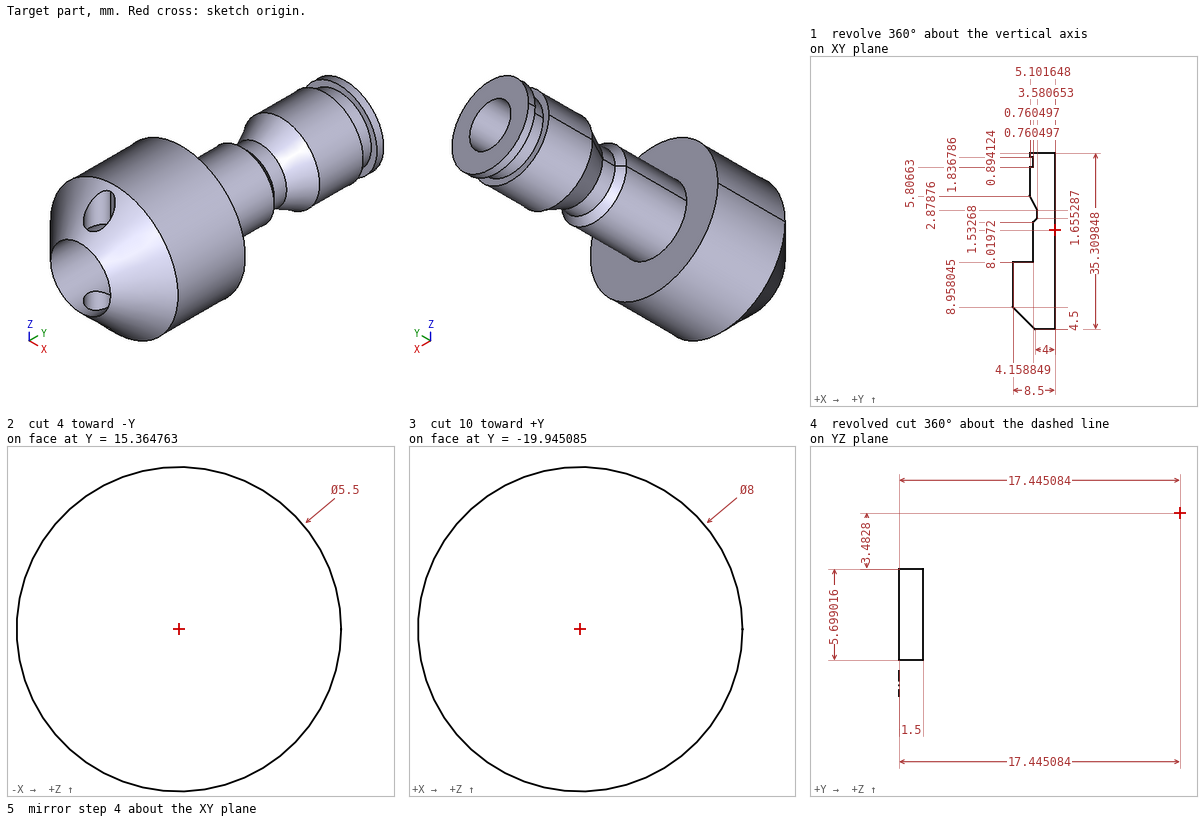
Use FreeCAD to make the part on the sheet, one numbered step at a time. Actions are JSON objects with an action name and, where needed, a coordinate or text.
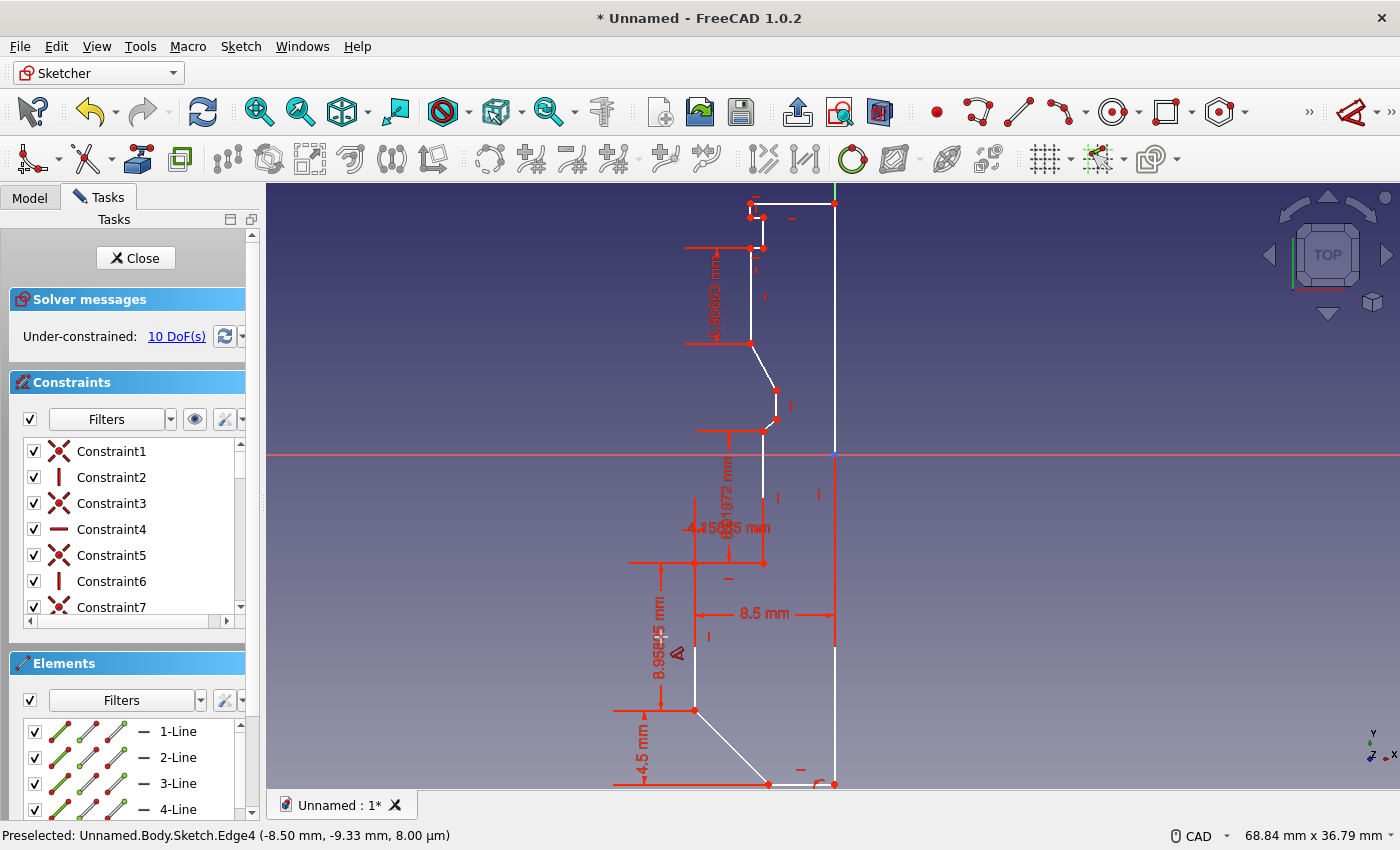
{"action": "scroll", "coordinate": [764, 472], "scroll_direction": "down", "scroll_amount": 2}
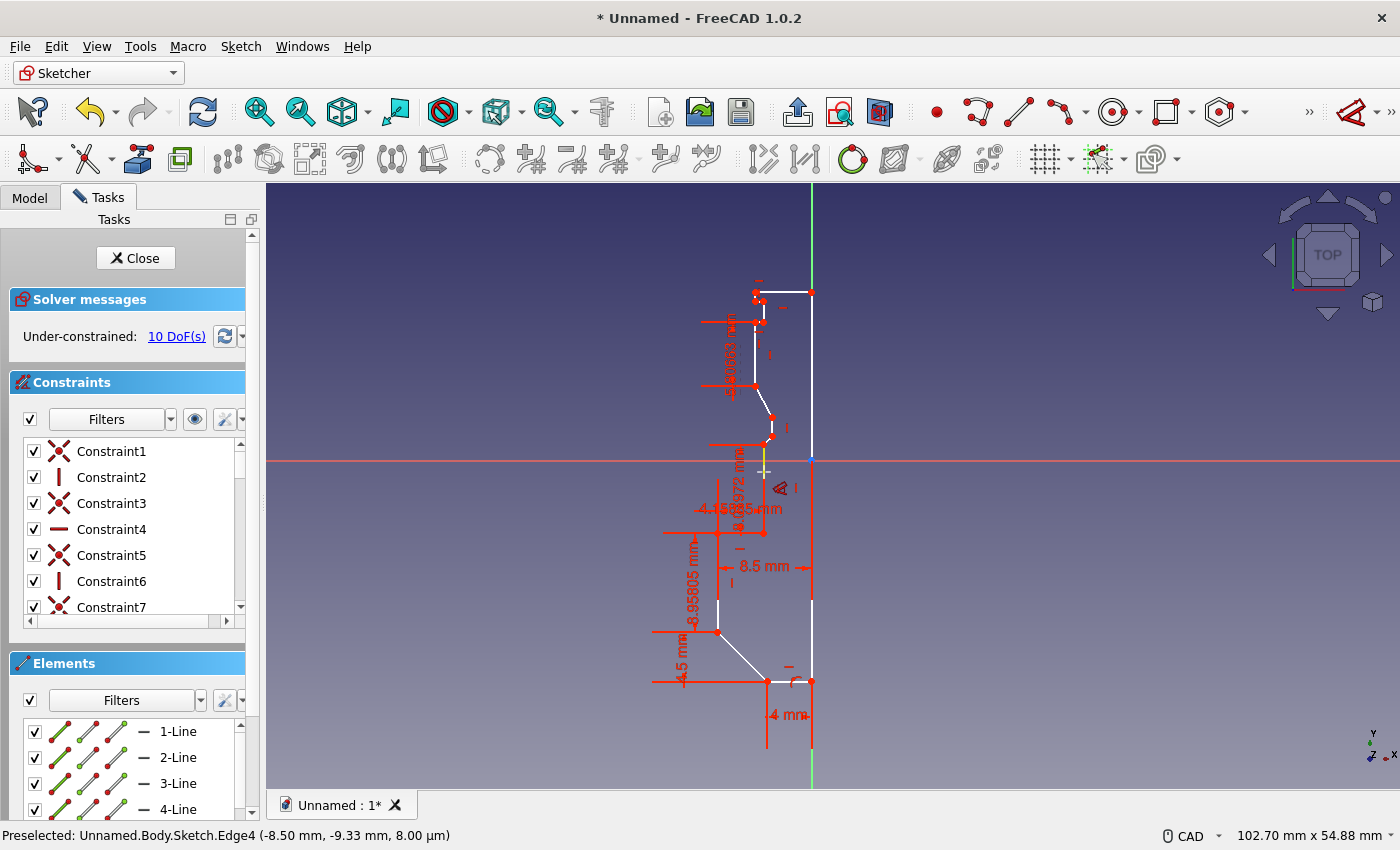
{"action": "left_click", "coordinate": [795, 292]}
{"action": "left_click", "coordinate": [783, 258]}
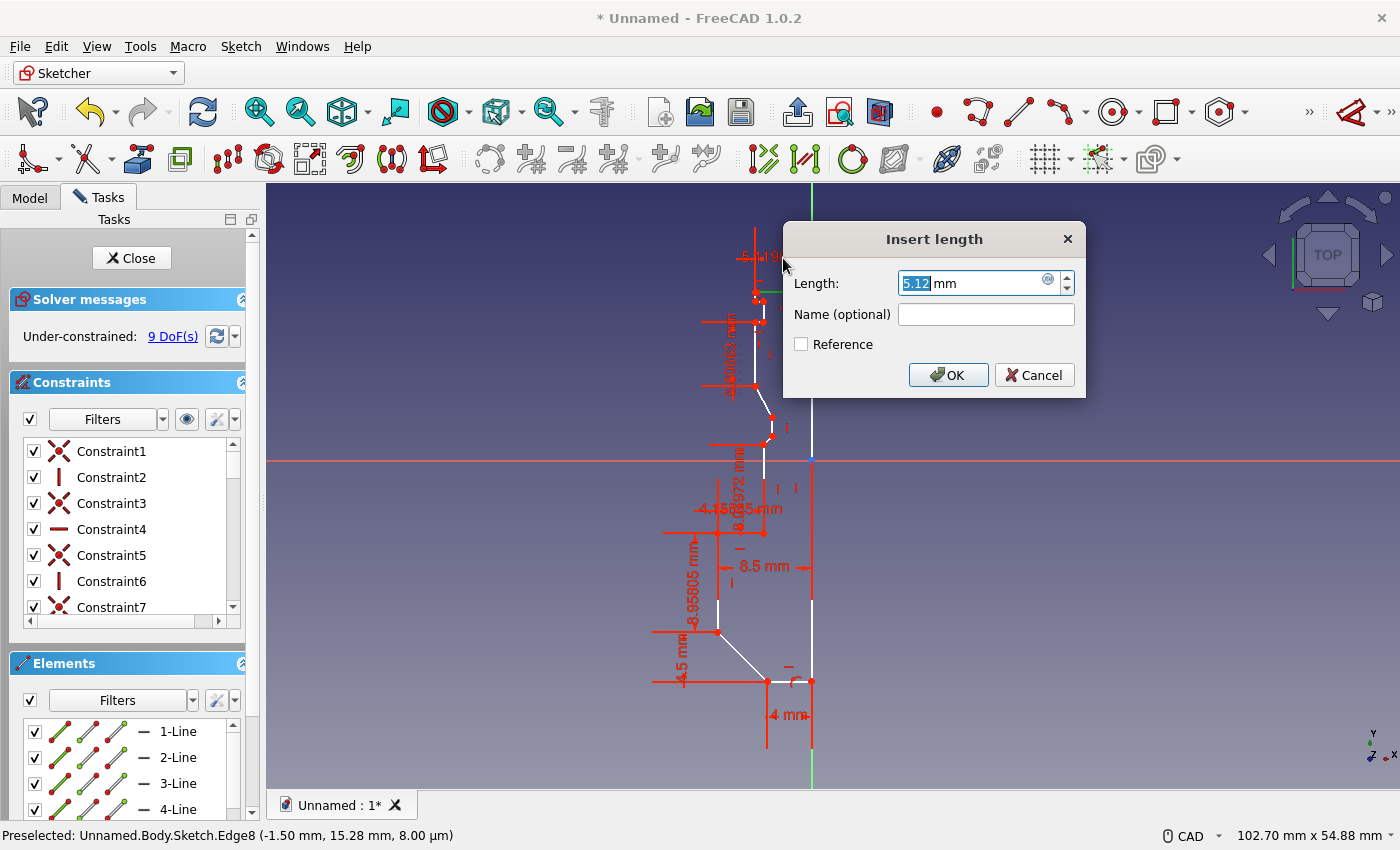
{"action": "type", "text": "5.101648"}
{"action": "key", "text": "Return"}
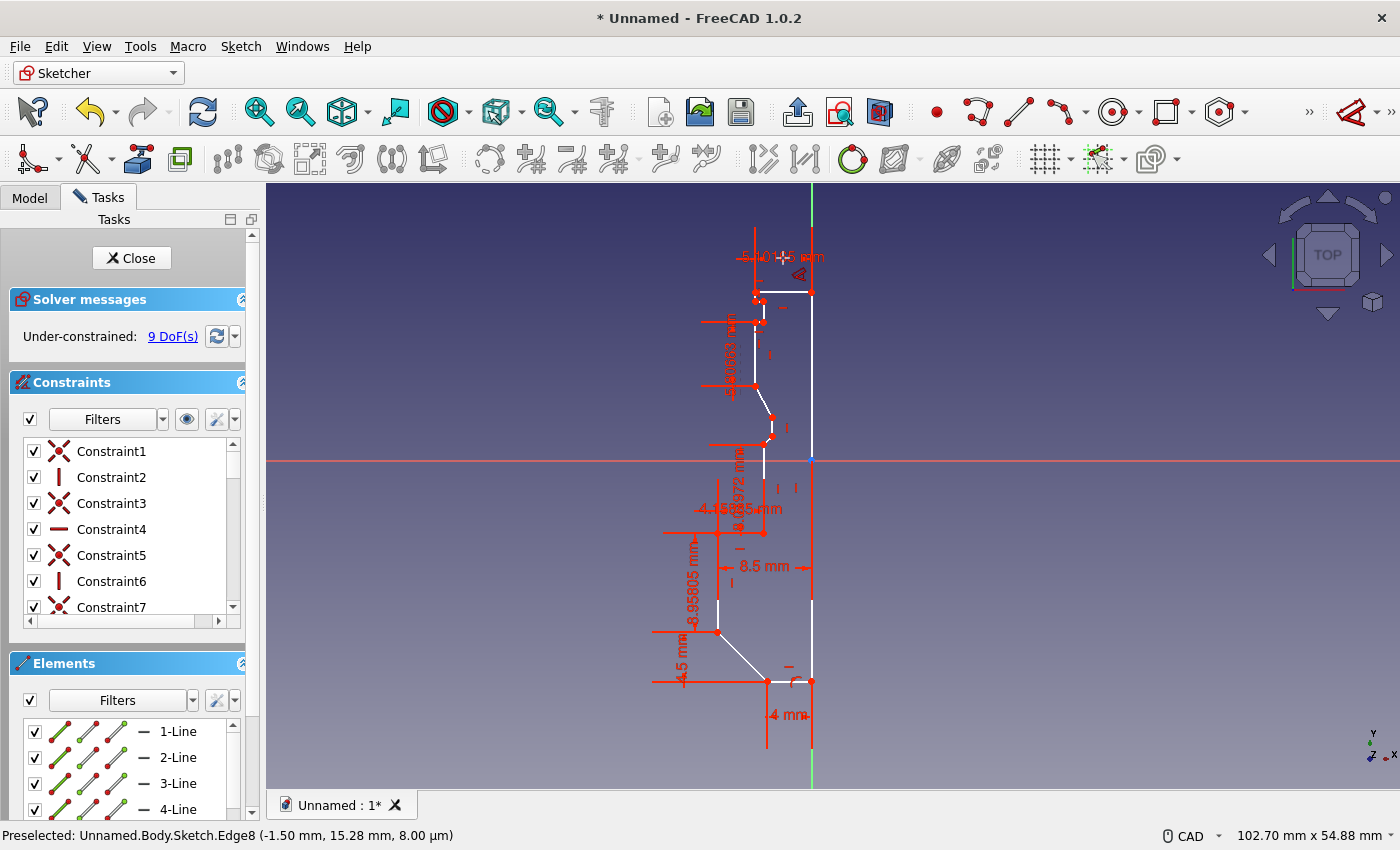
{"action": "scroll", "coordinate": [755, 297], "scroll_direction": "up", "scroll_amount": 7}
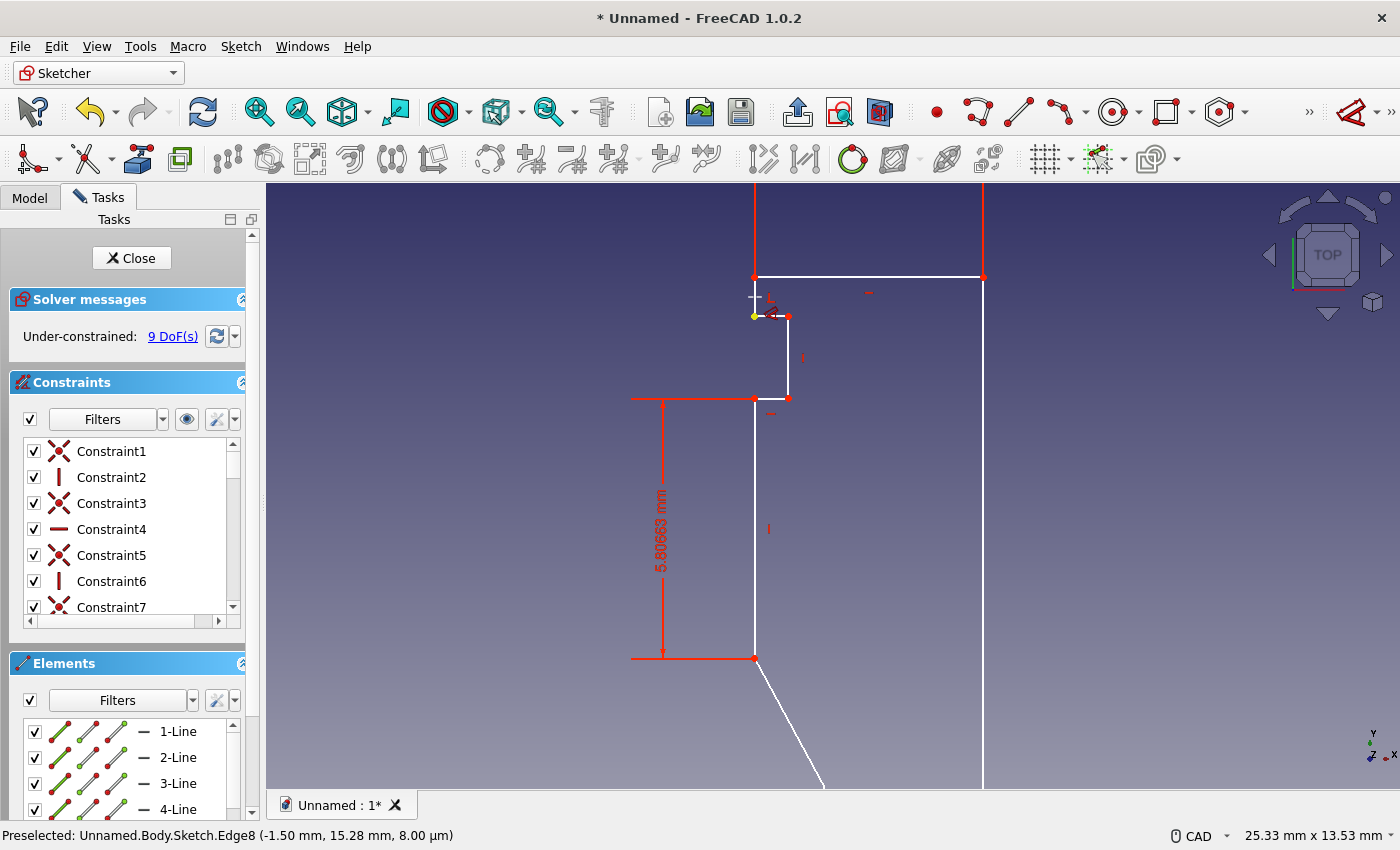
{"action": "left_click", "coordinate": [755, 297]}
{"action": "left_click", "coordinate": [721, 297]}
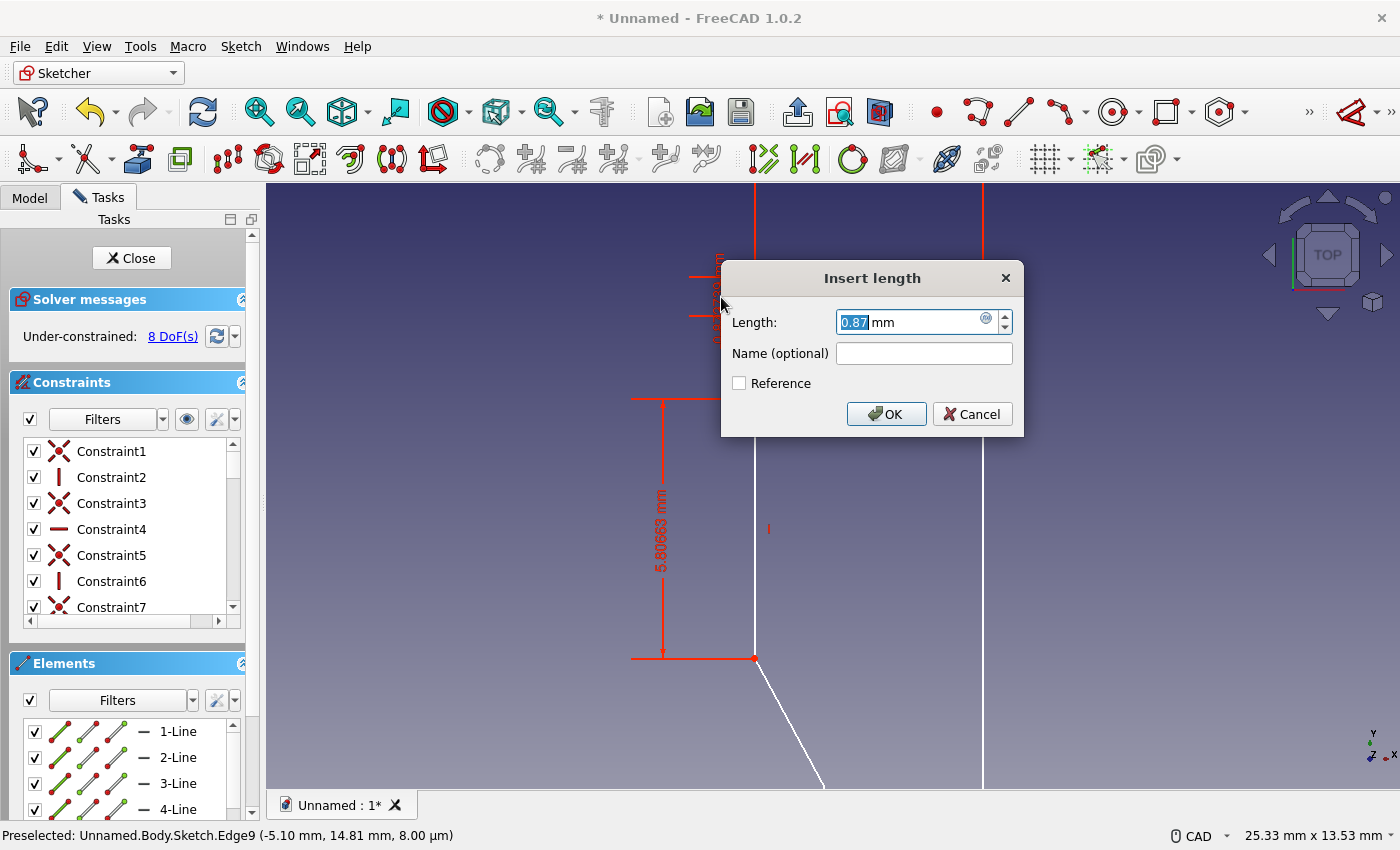
{"action": "type", "text": "0.894124"}
{"action": "key", "text": "Return"}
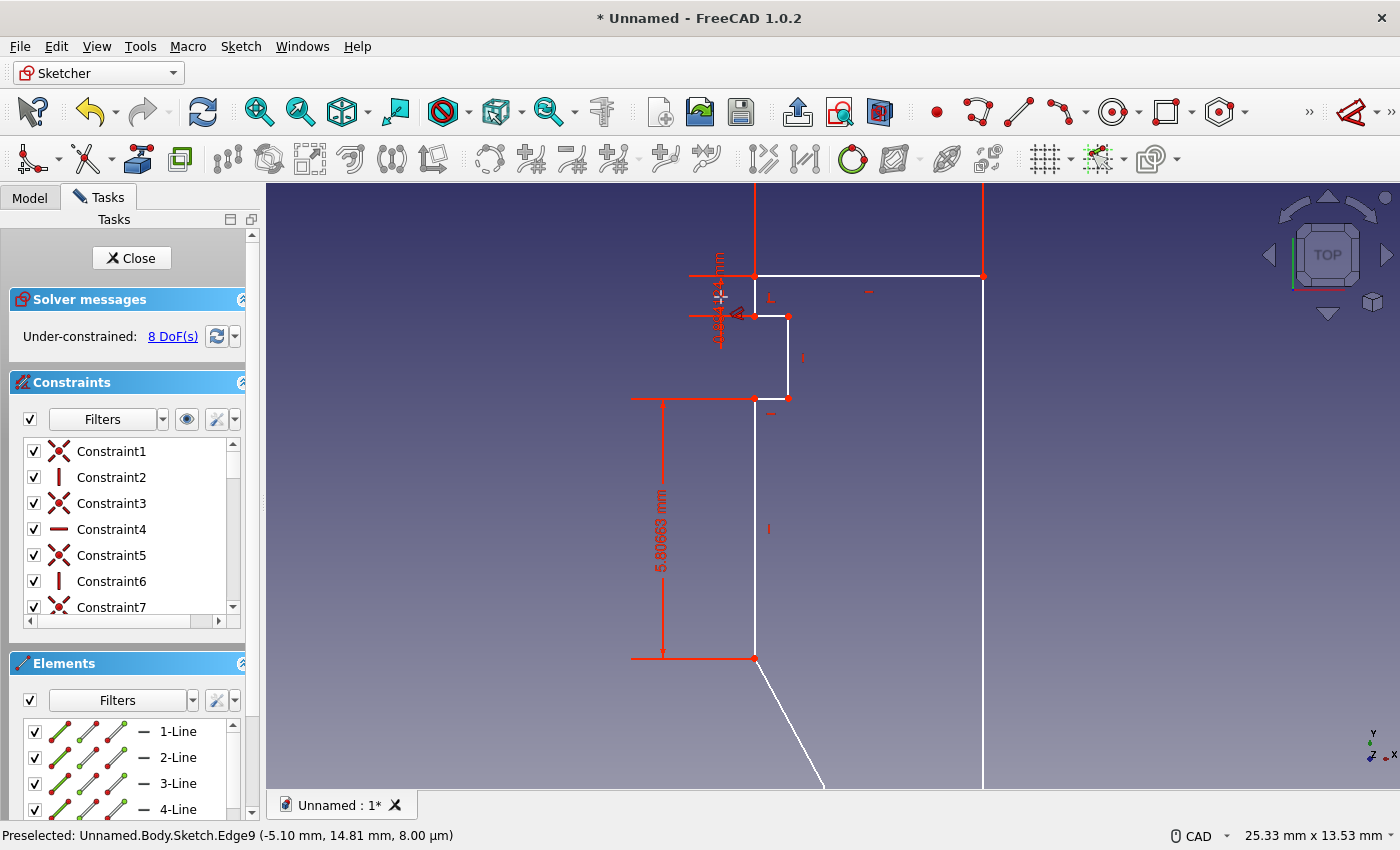
{"action": "scroll", "coordinate": [765, 316], "scroll_direction": "up", "scroll_amount": 2}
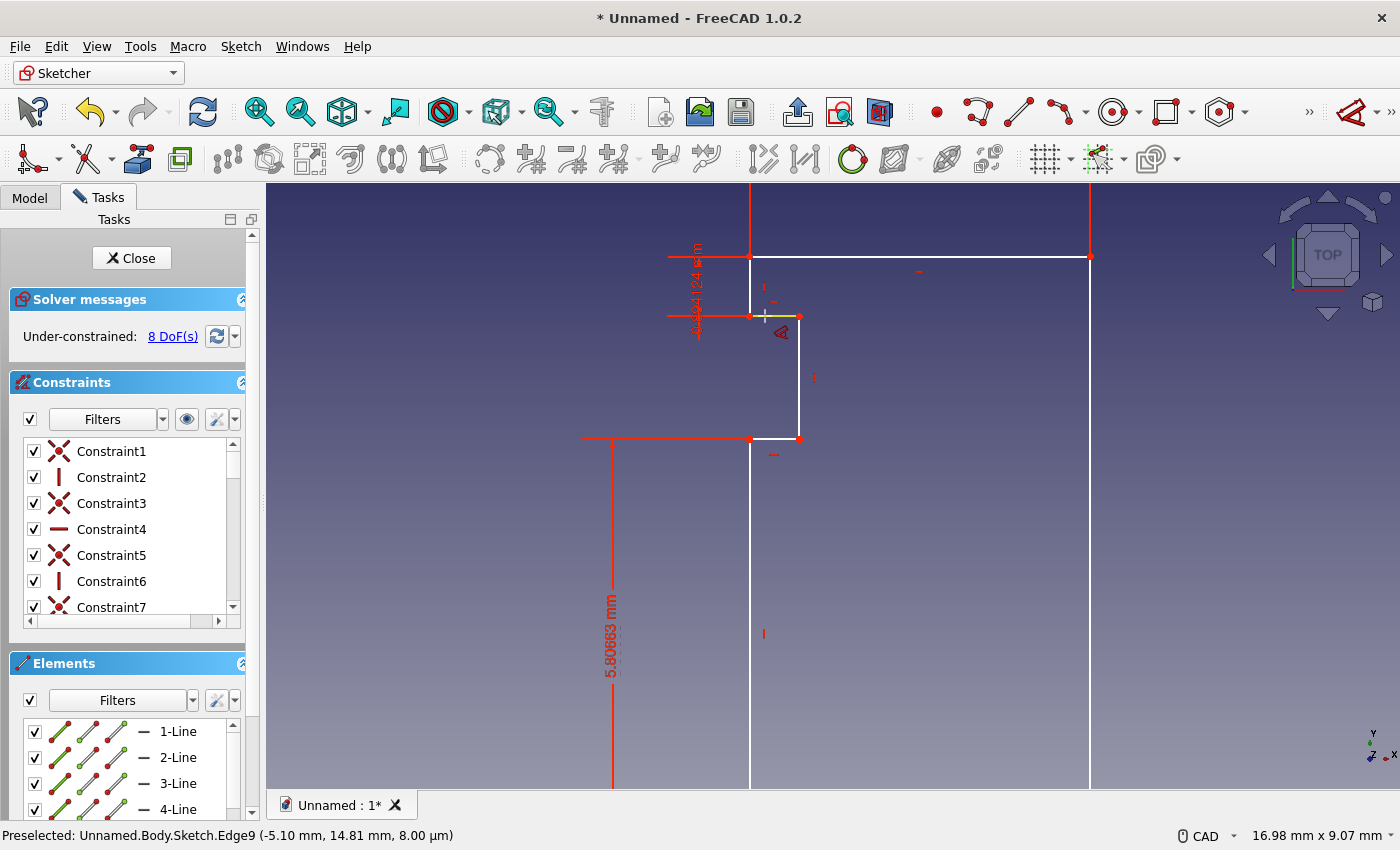
{"action": "left_click", "coordinate": [764, 316]}
{"action": "left_click", "coordinate": [774, 282]}